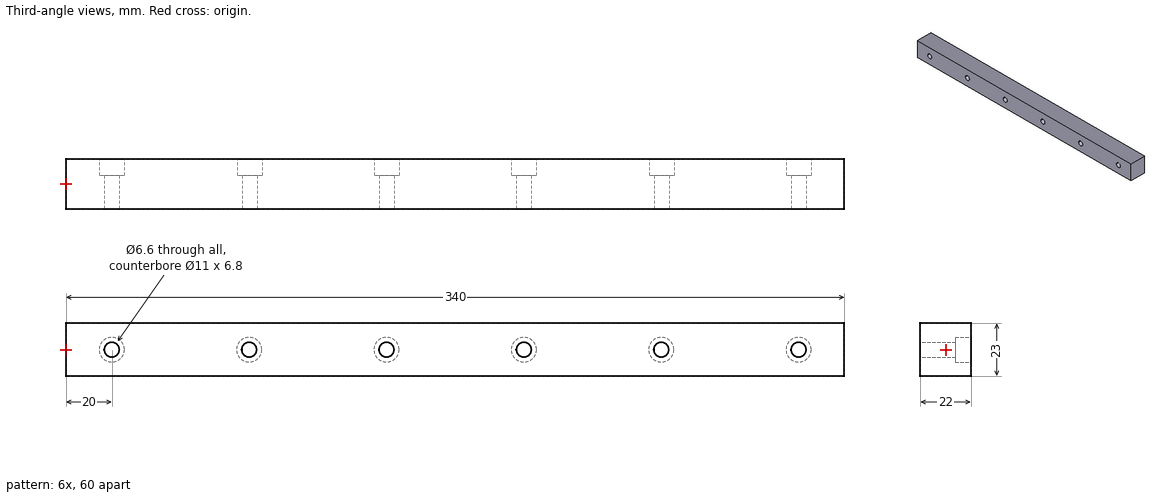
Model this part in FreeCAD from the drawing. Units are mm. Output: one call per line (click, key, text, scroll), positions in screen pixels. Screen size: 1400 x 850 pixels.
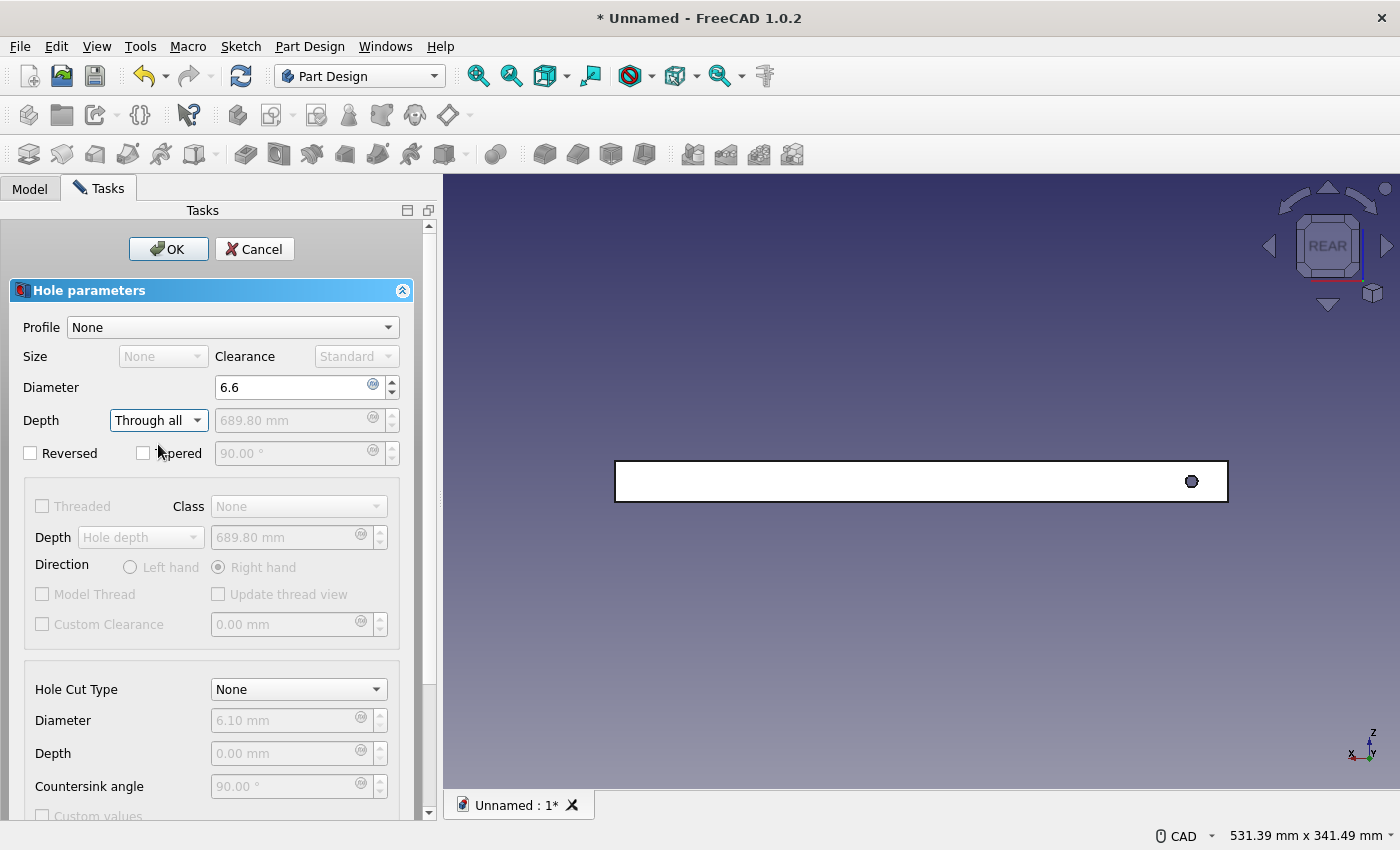
click(300, 690)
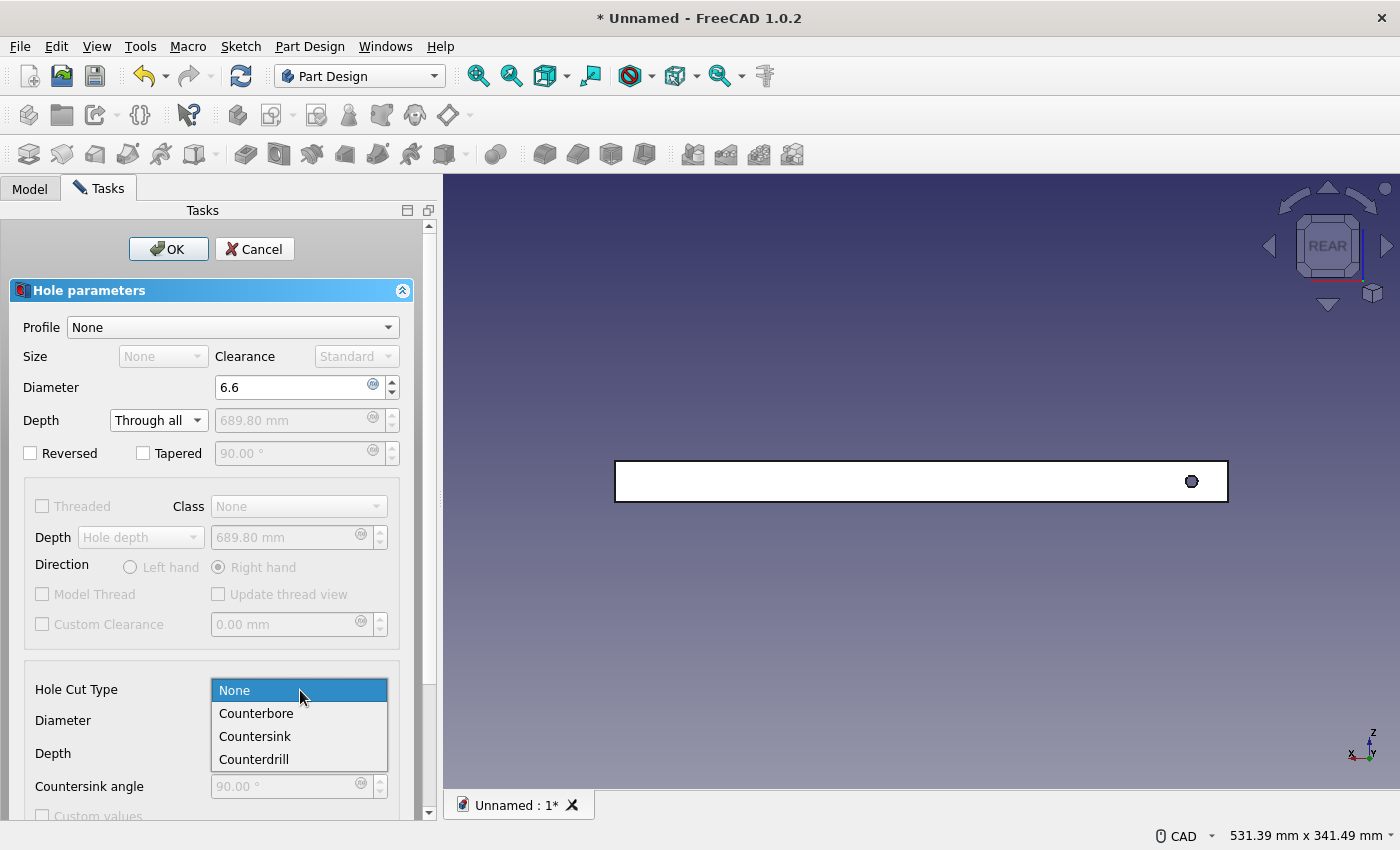
click(298, 714)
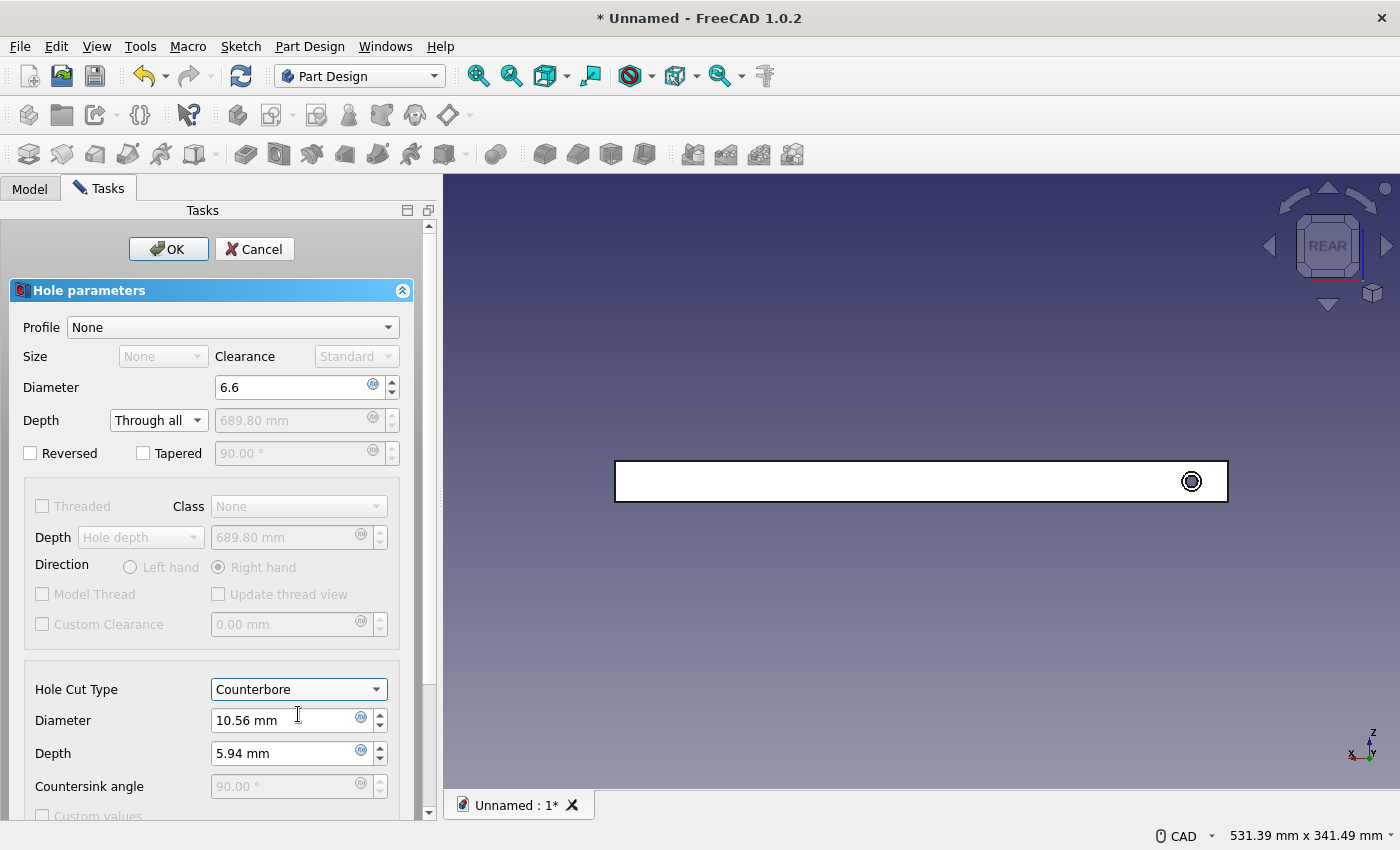
triple_click(292, 720)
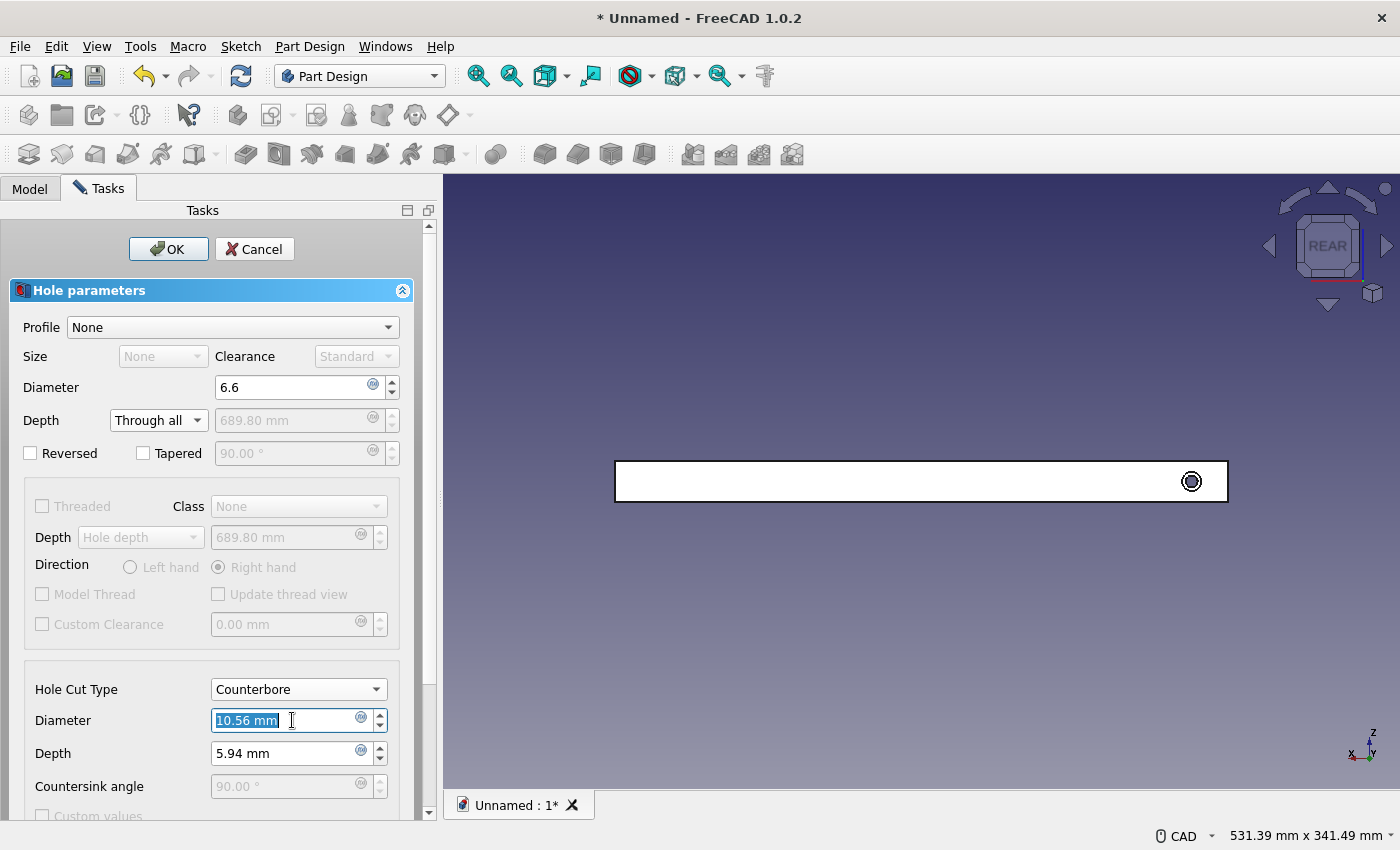
text(11)
key(Tab)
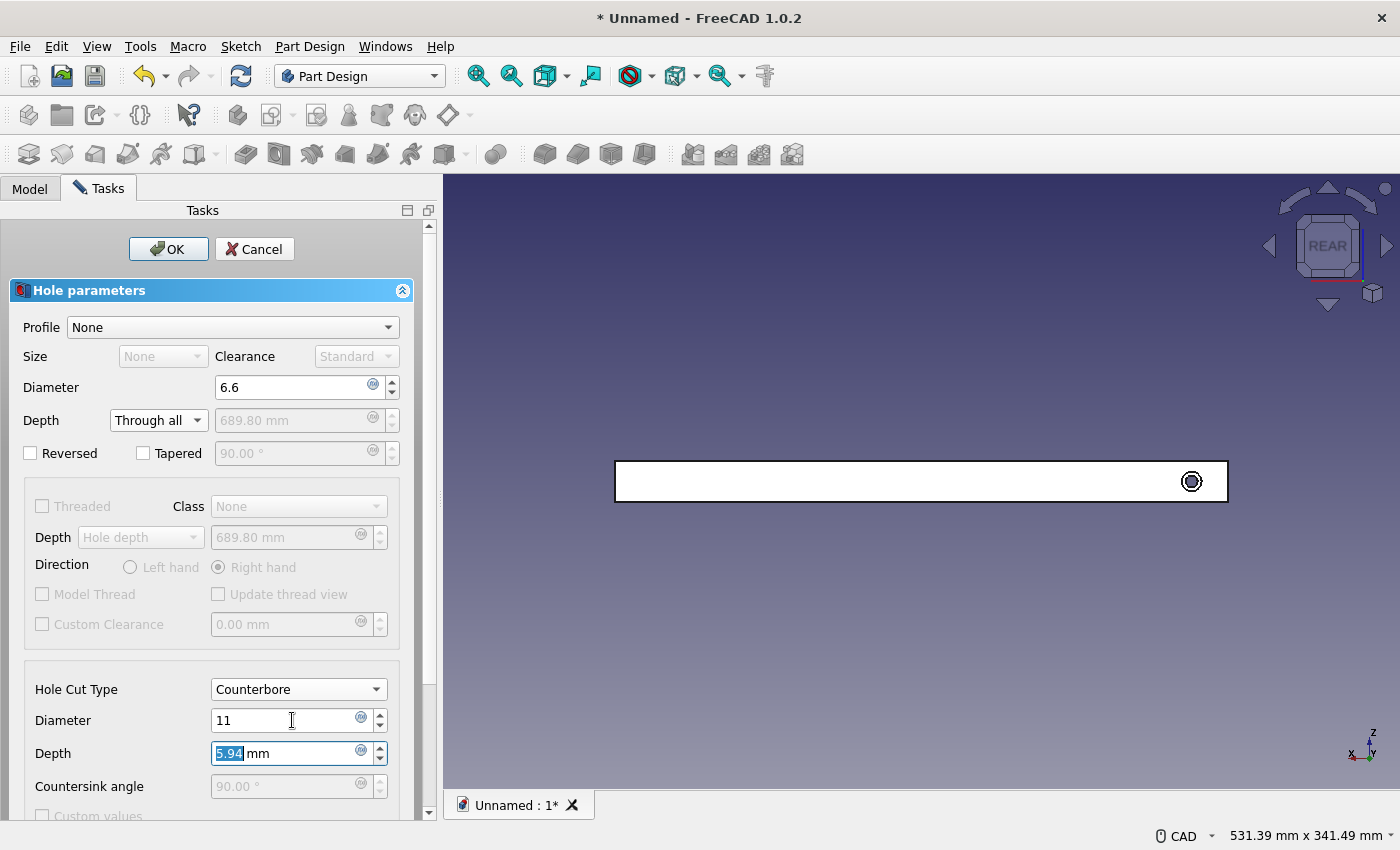
text(6.8)
key(Tab)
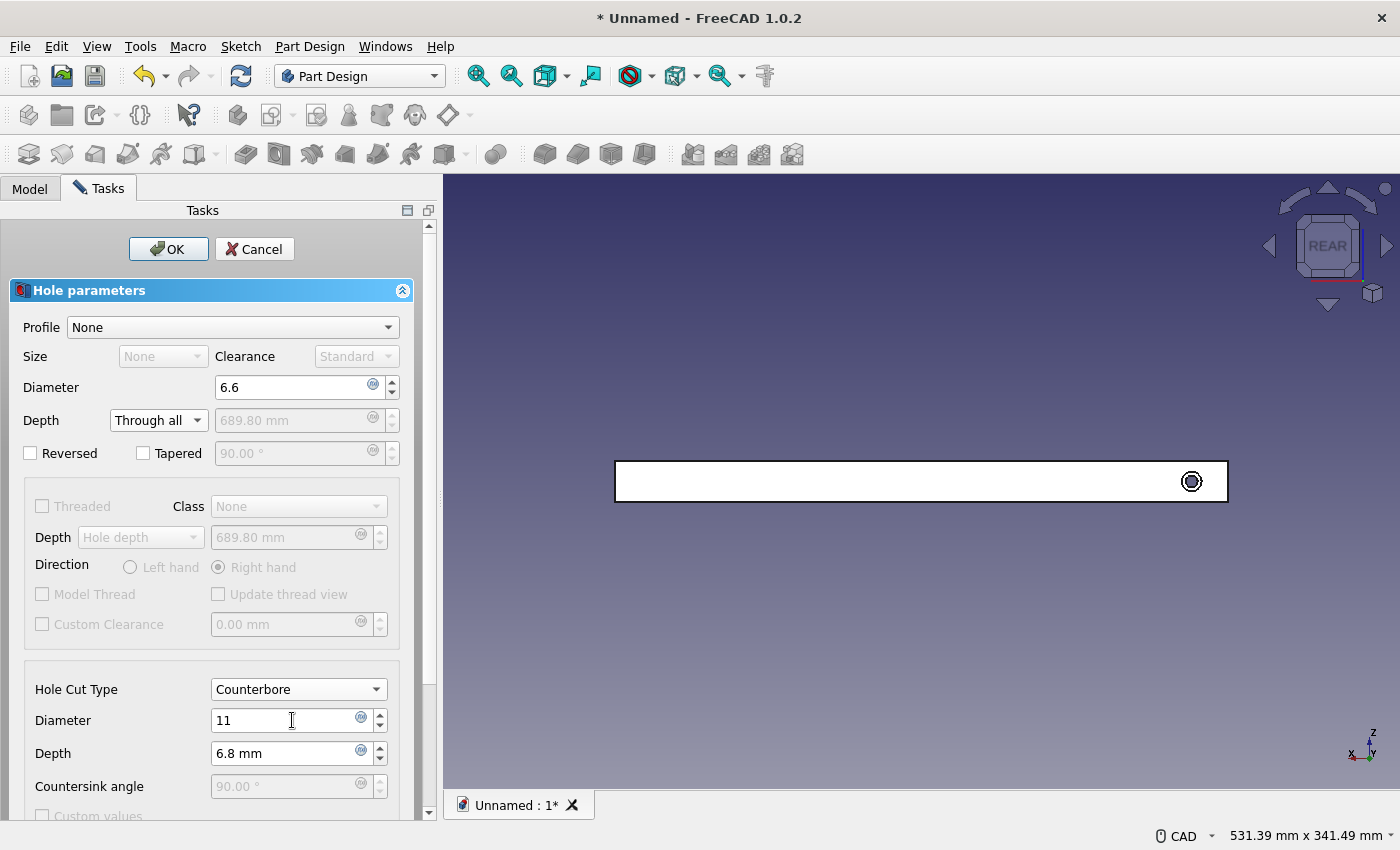
click(169, 249)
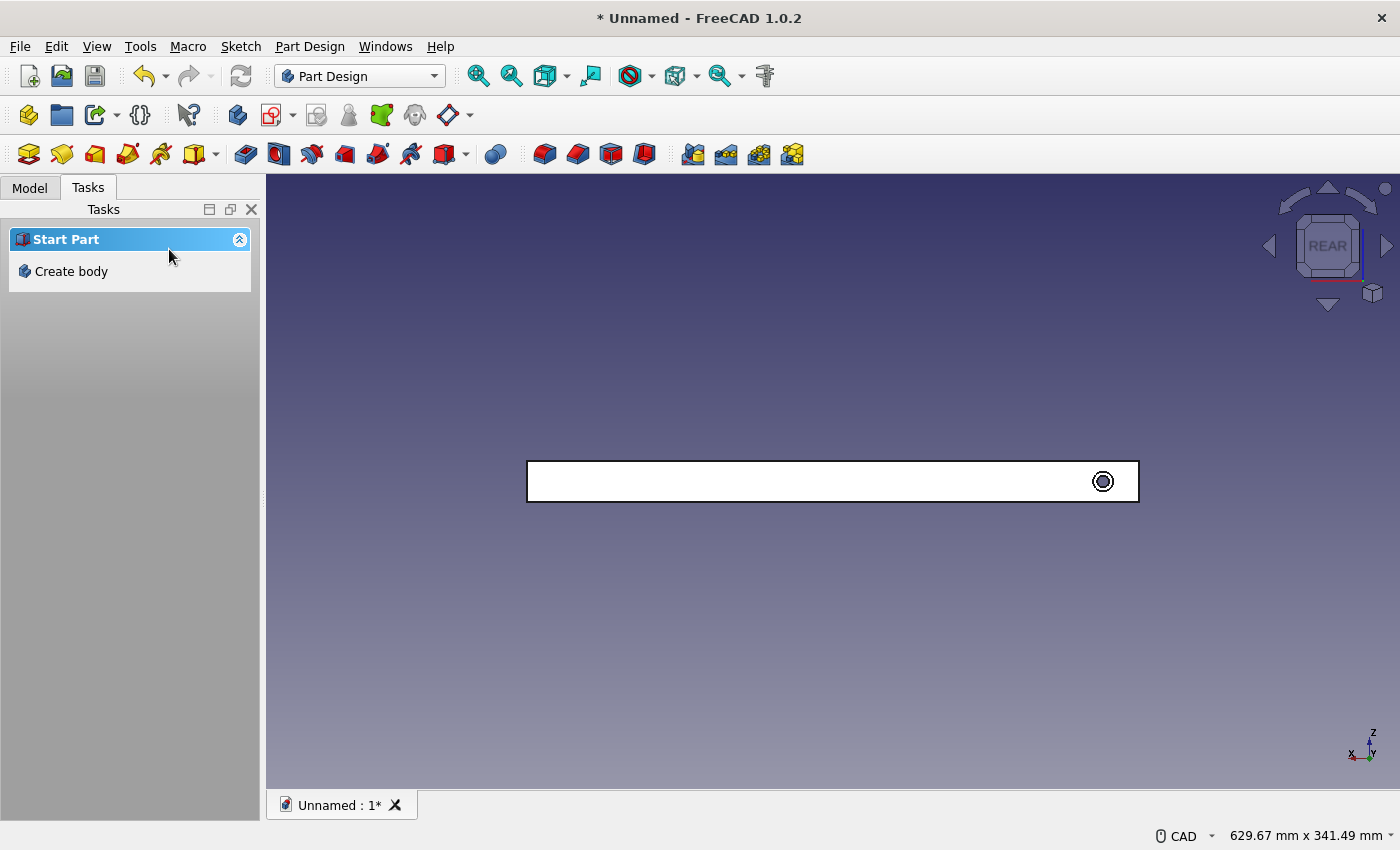
click(30, 188)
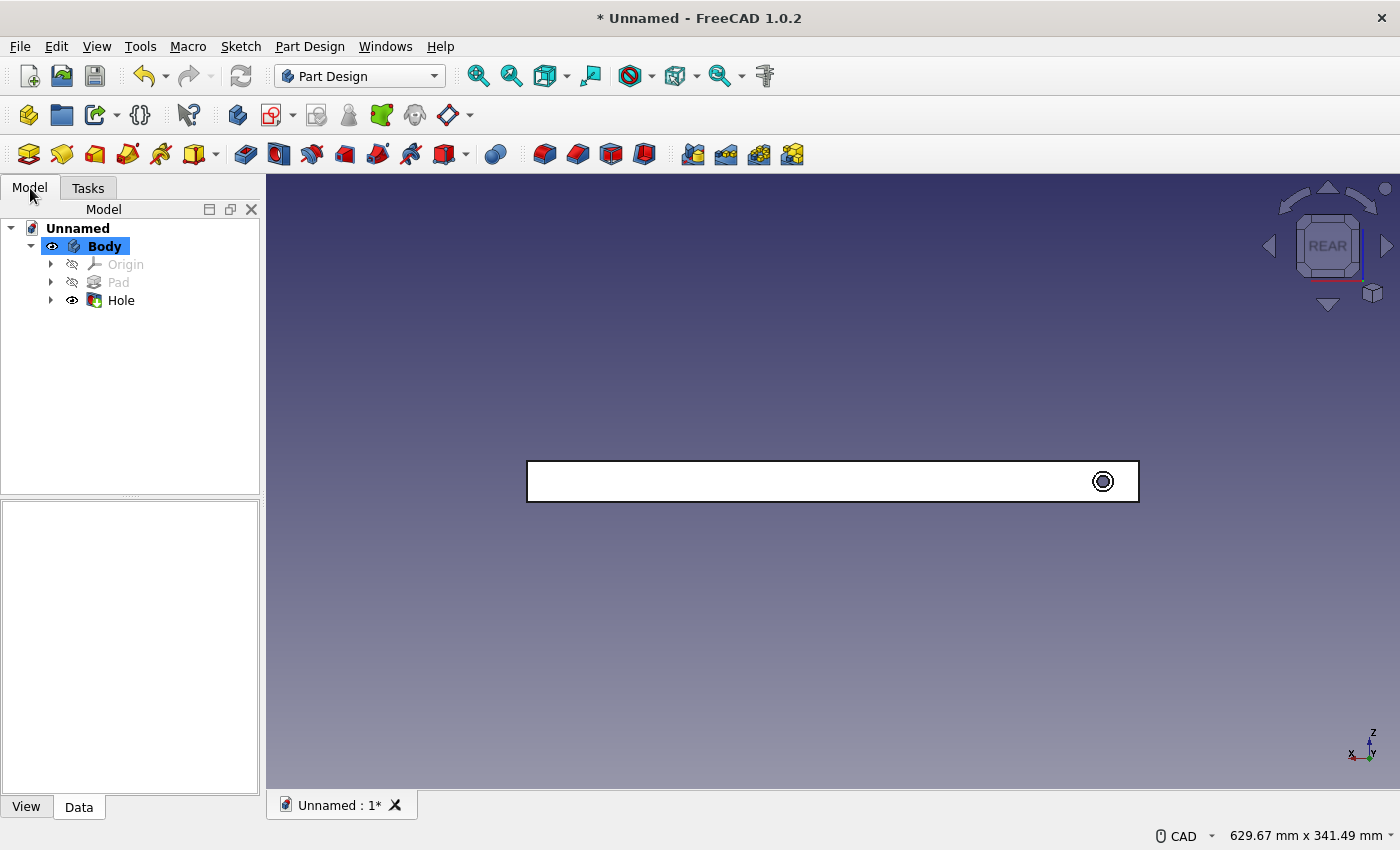
click(117, 300)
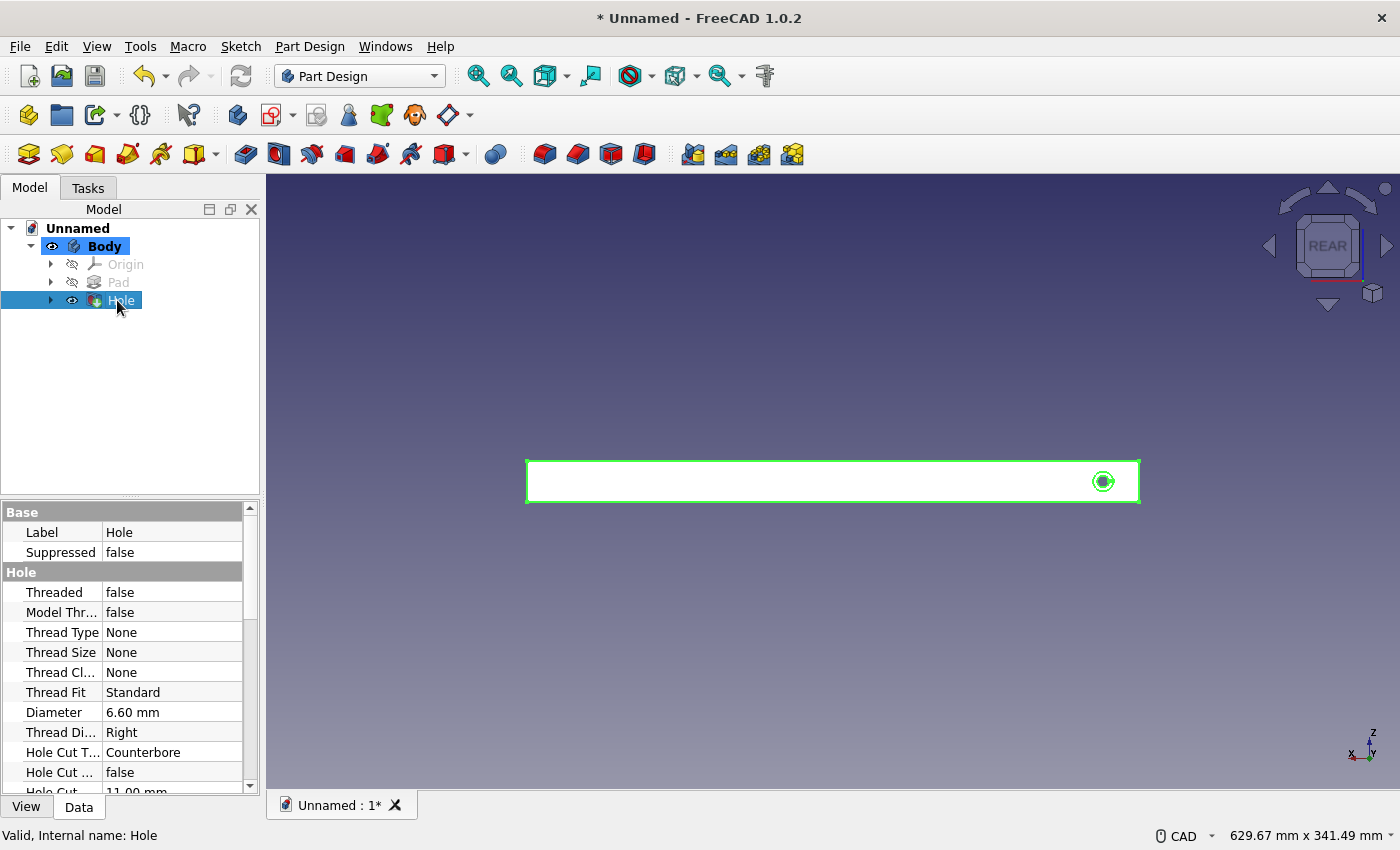
click(726, 154)